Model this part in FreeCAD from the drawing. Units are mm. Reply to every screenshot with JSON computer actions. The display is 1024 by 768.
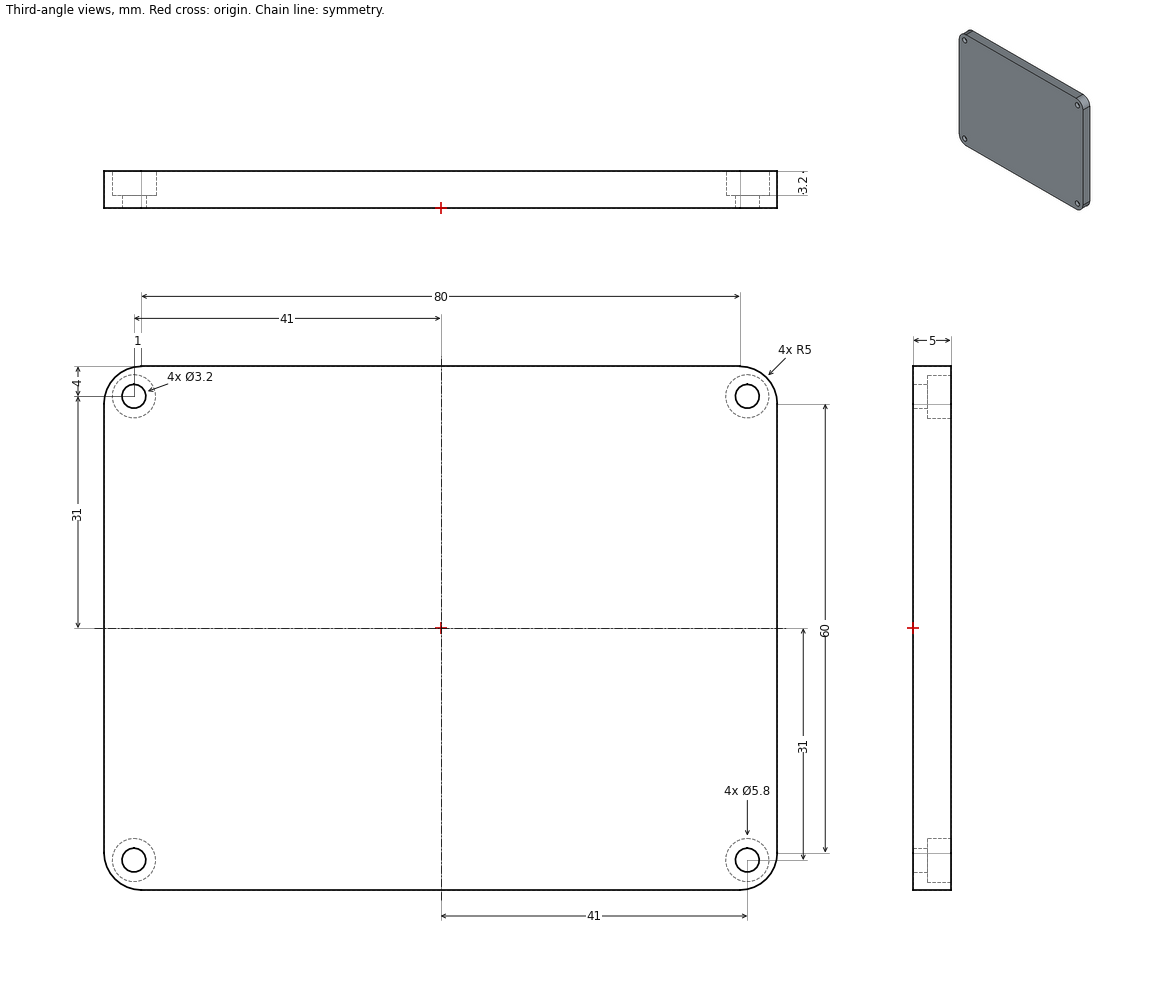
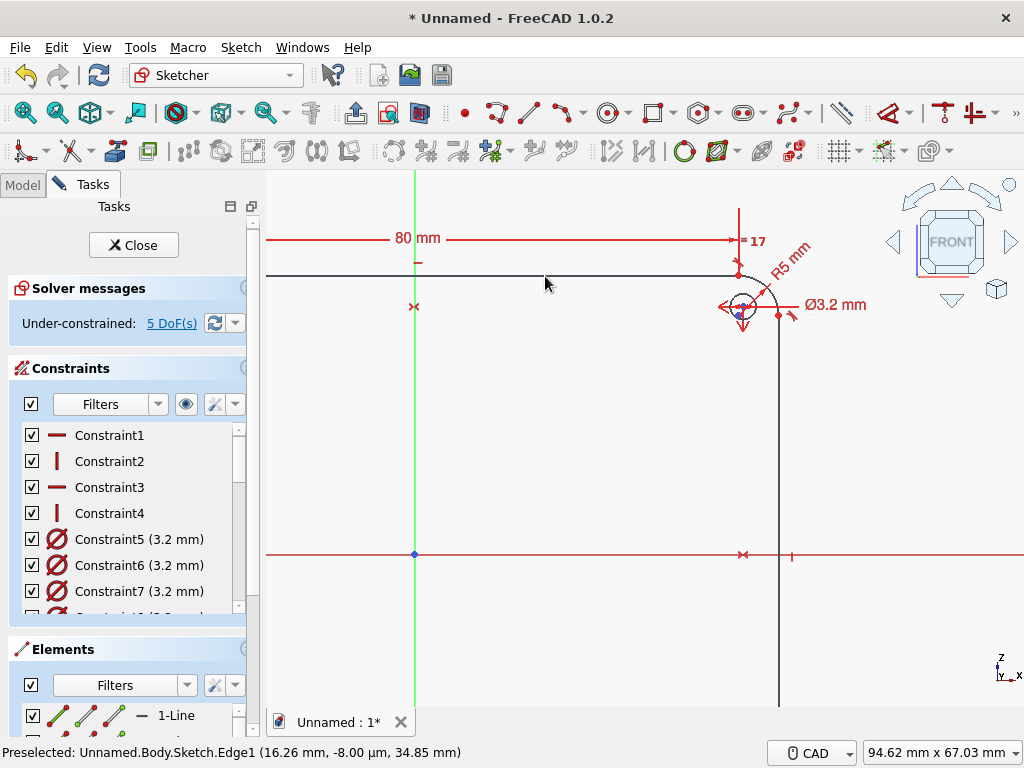
{"action": "left_click", "coordinate": [779, 460]}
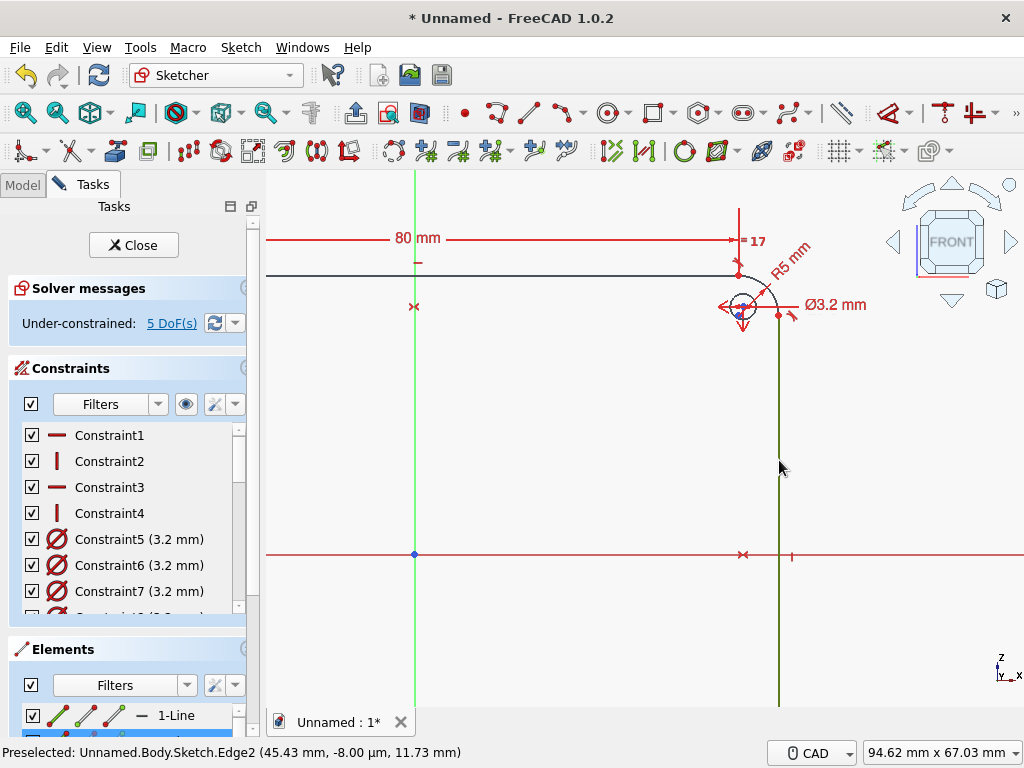
{"action": "key", "text": "i"}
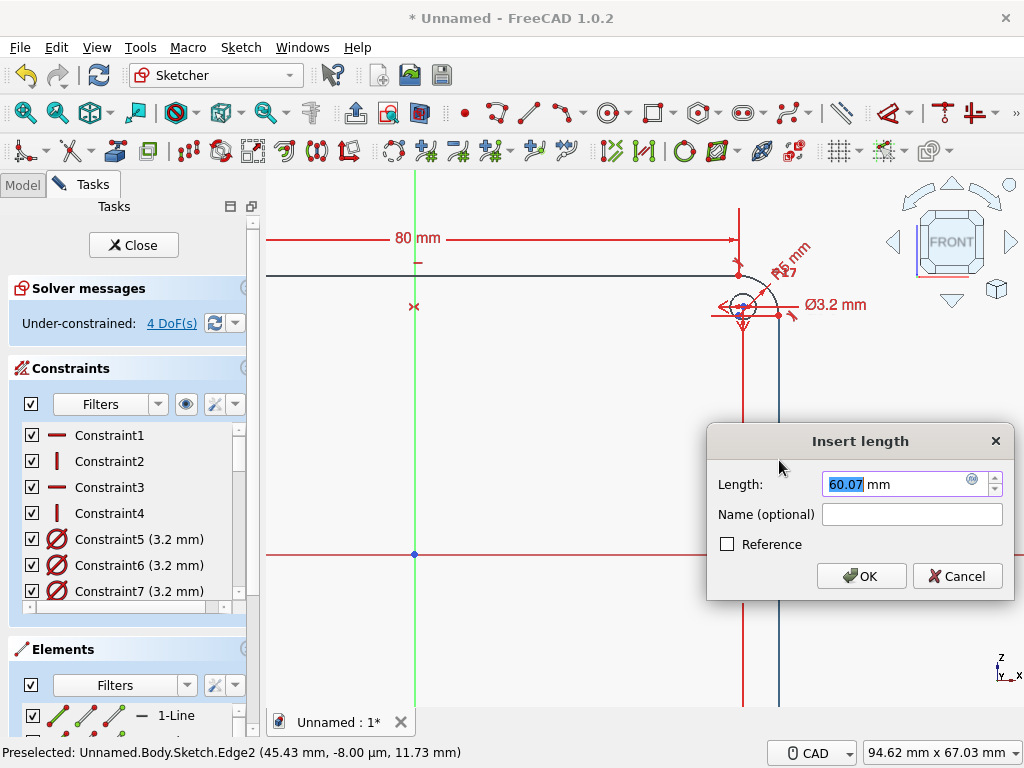
{"action": "type", "text": "60"}
{"action": "key", "text": "Return"}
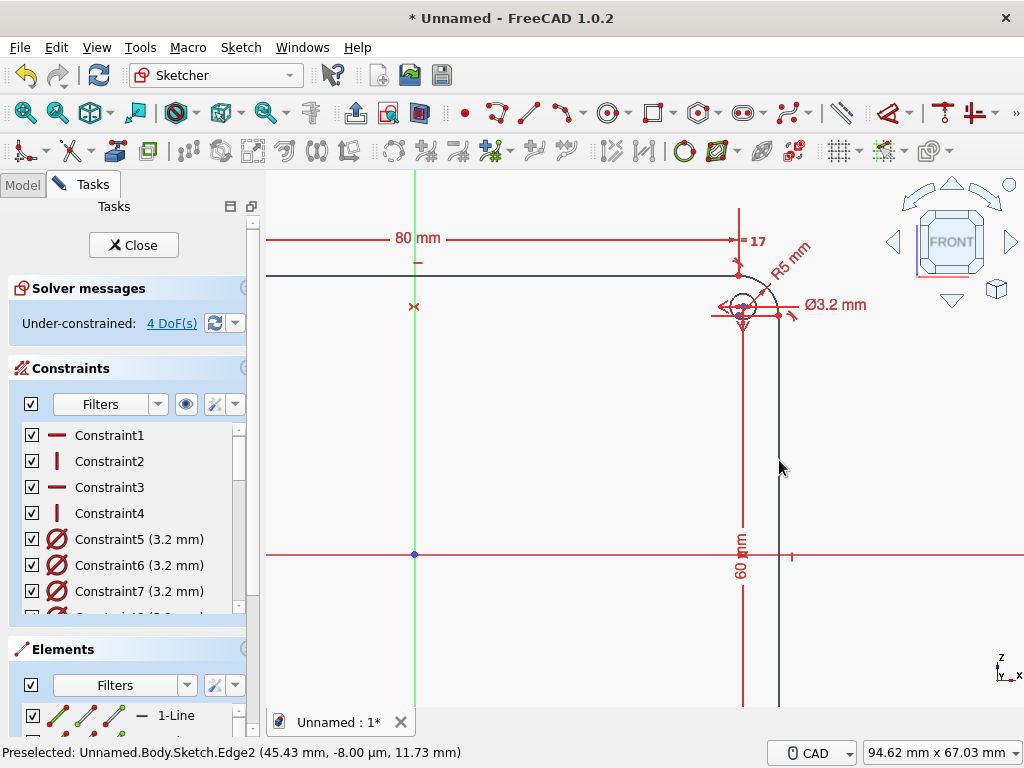
{"action": "scroll", "coordinate": [773, 297], "scroll_direction": "down", "scroll_amount": 3}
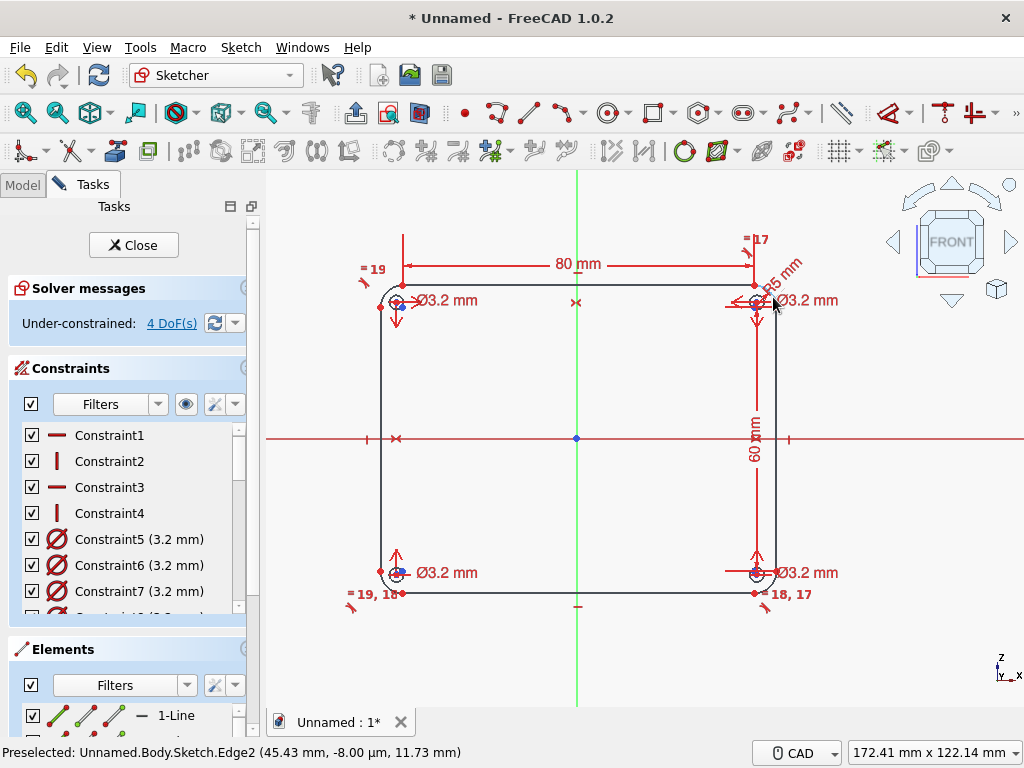
{"action": "scroll", "coordinate": [396, 302], "scroll_direction": "up", "scroll_amount": 3}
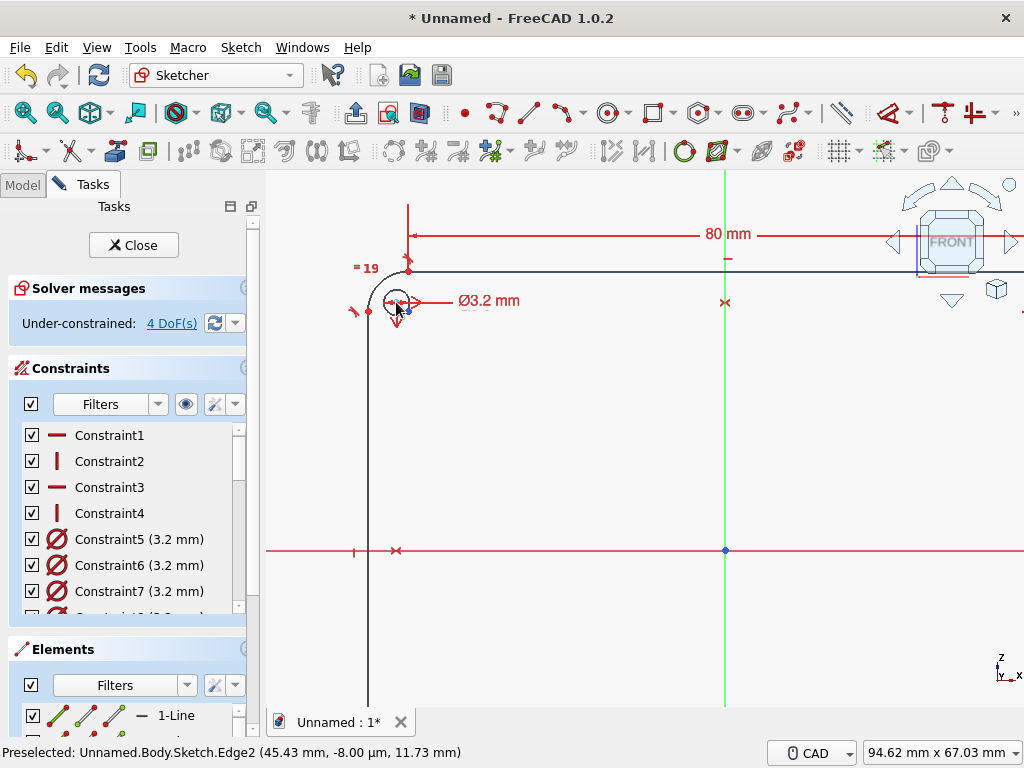
{"action": "left_click", "coordinate": [397, 303]}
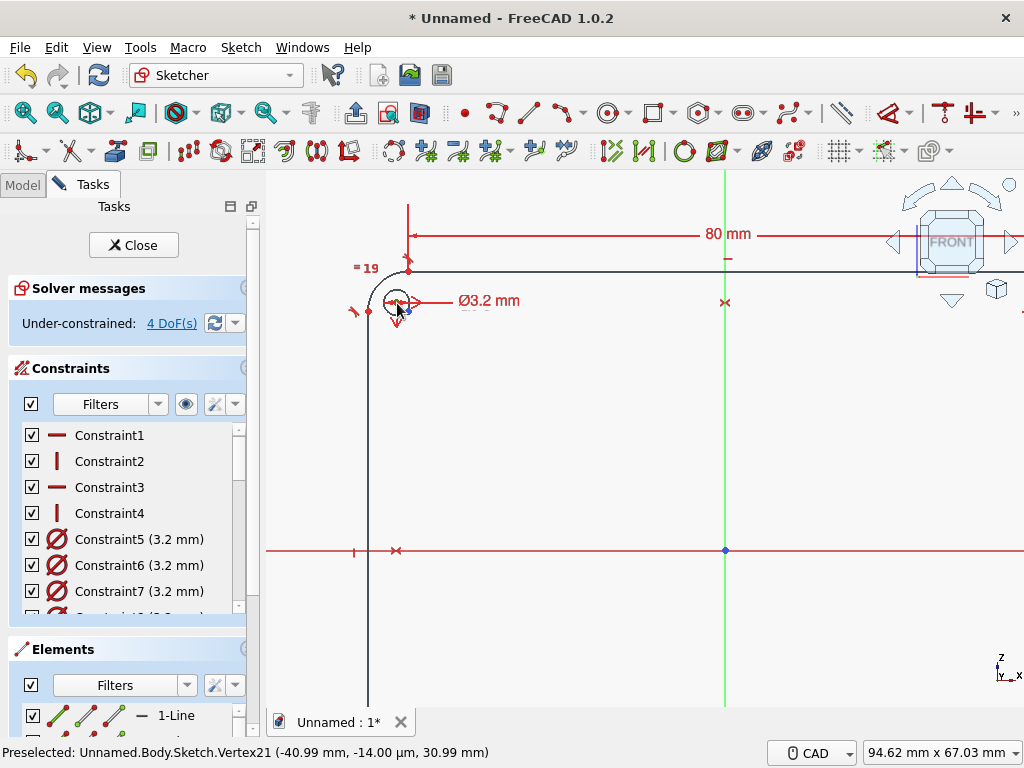
{"action": "left_click", "coordinate": [912, 114]}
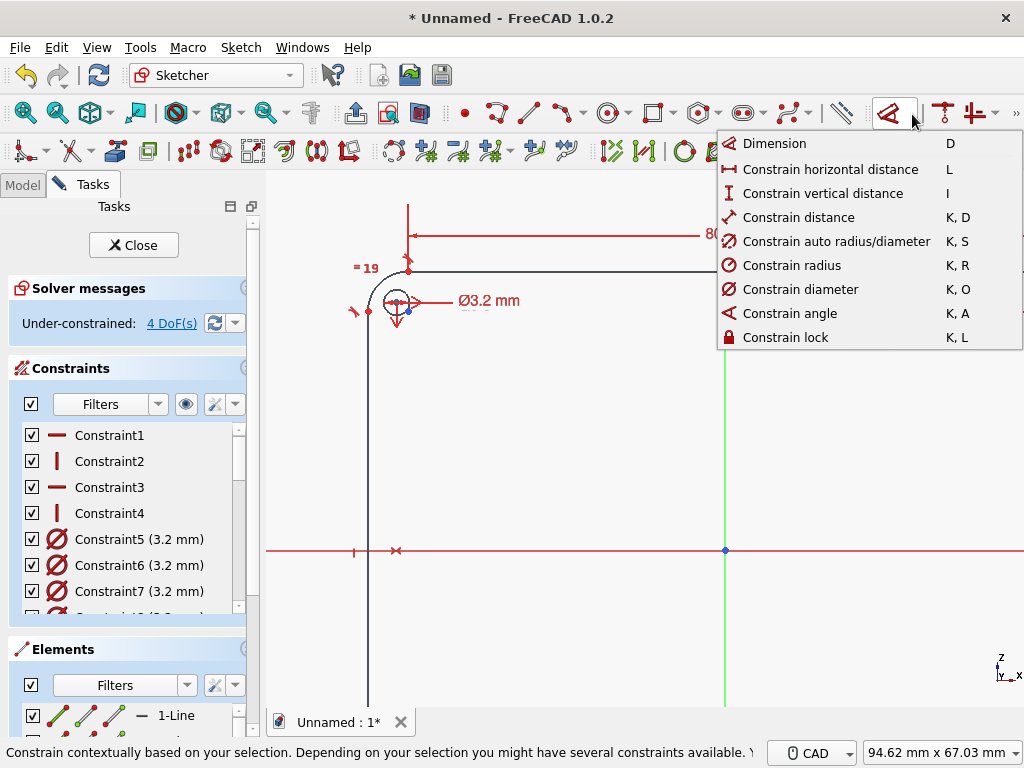
{"action": "left_click", "coordinate": [870, 169]}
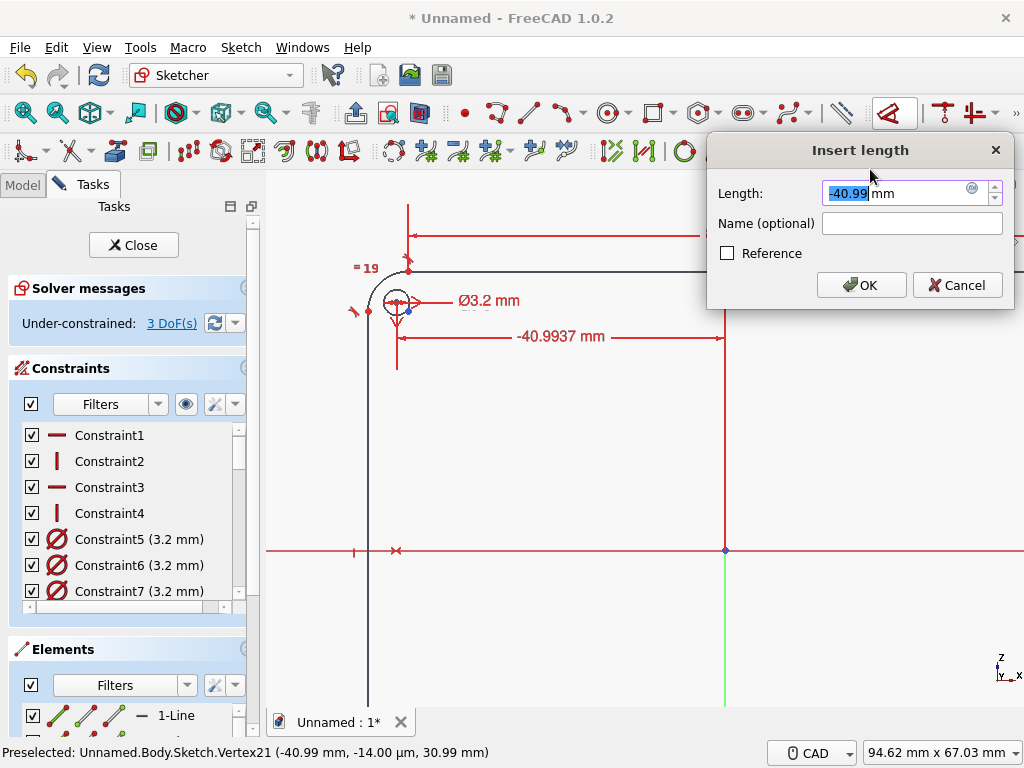
{"action": "type", "text": "-41"}
{"action": "key", "text": "Return"}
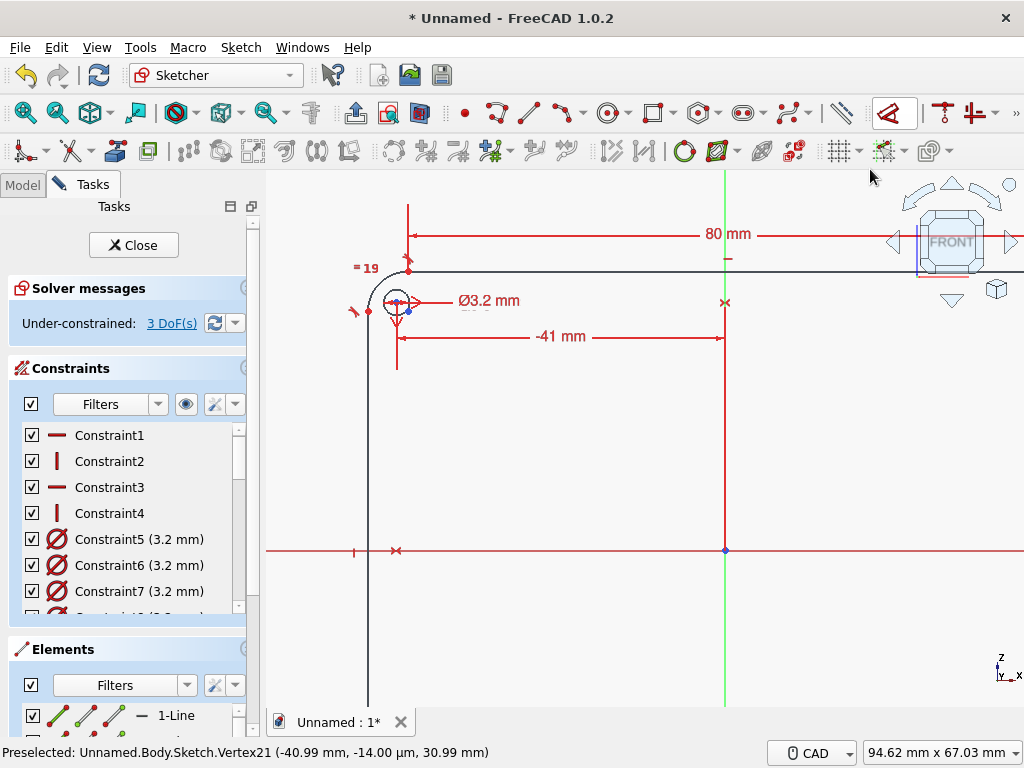
{"action": "left_click", "coordinate": [397, 303]}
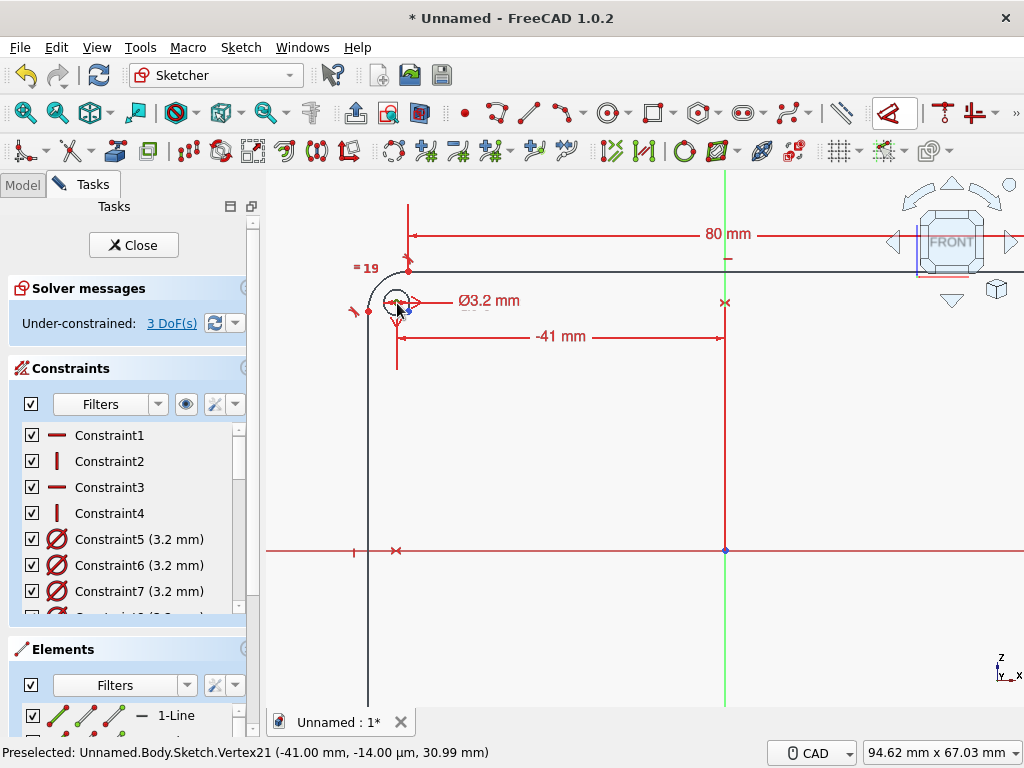
{"action": "key", "text": "i"}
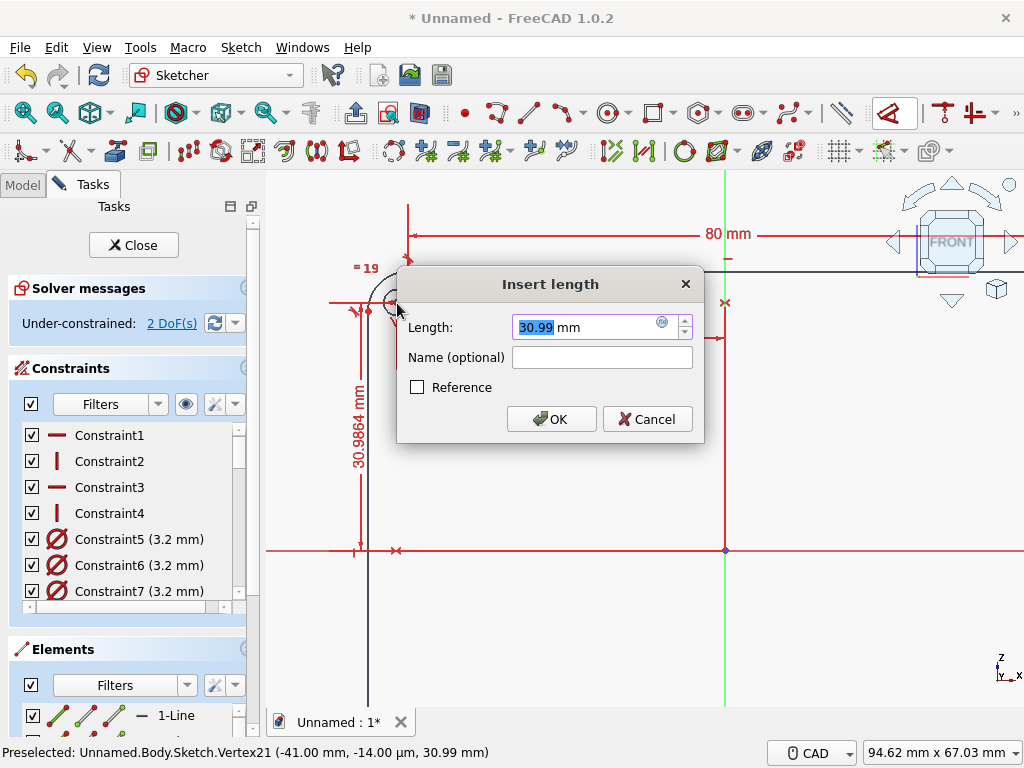
{"action": "type", "text": "31"}
{"action": "key", "text": "Return"}